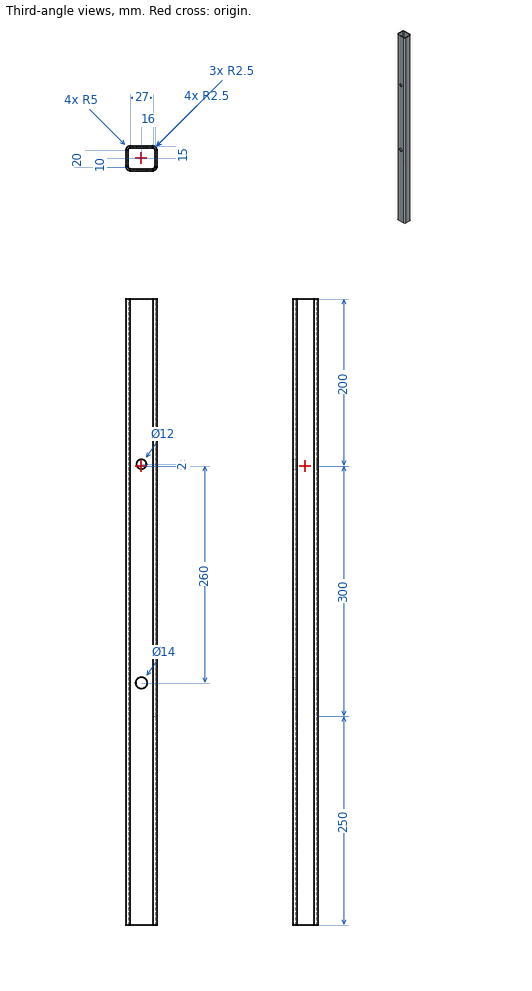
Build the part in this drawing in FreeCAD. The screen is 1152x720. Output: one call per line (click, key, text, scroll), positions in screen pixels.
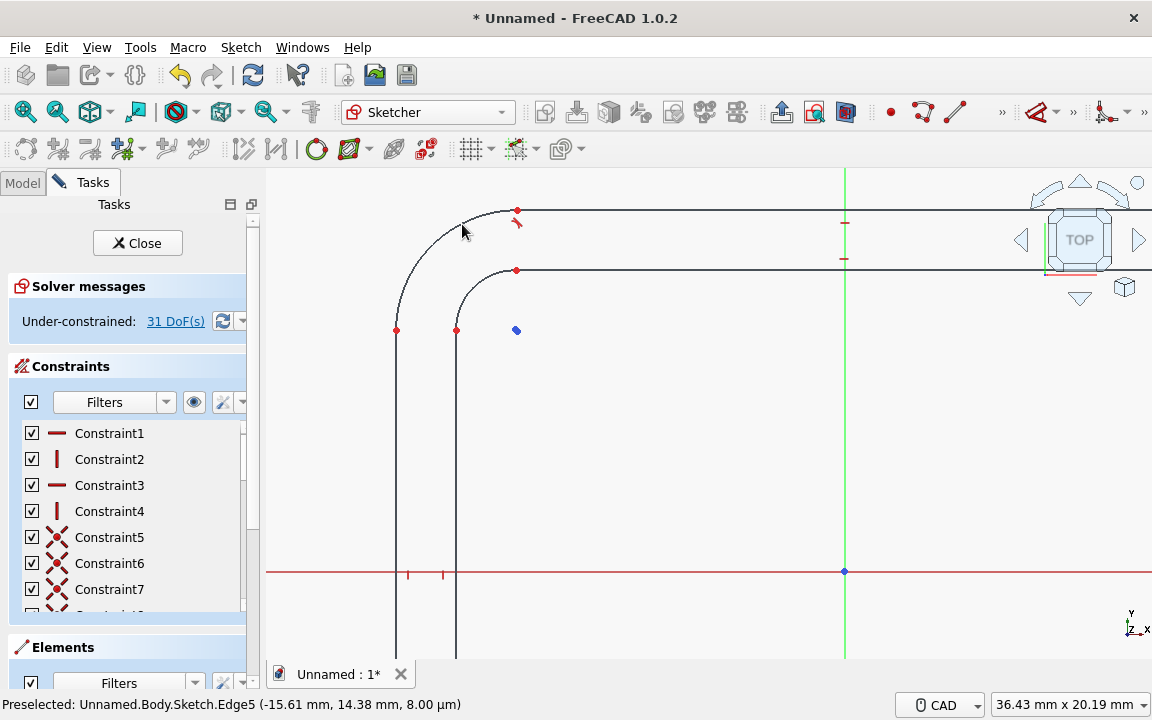
click(976, 210)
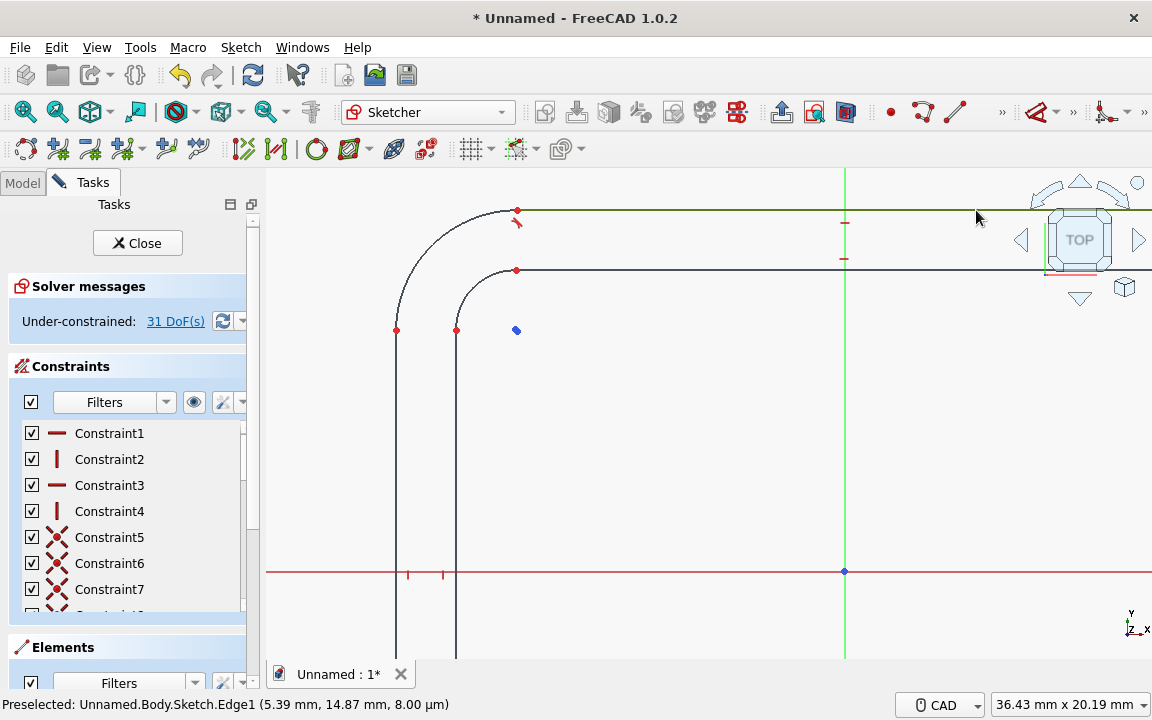
scroll(474, 284, down, 4)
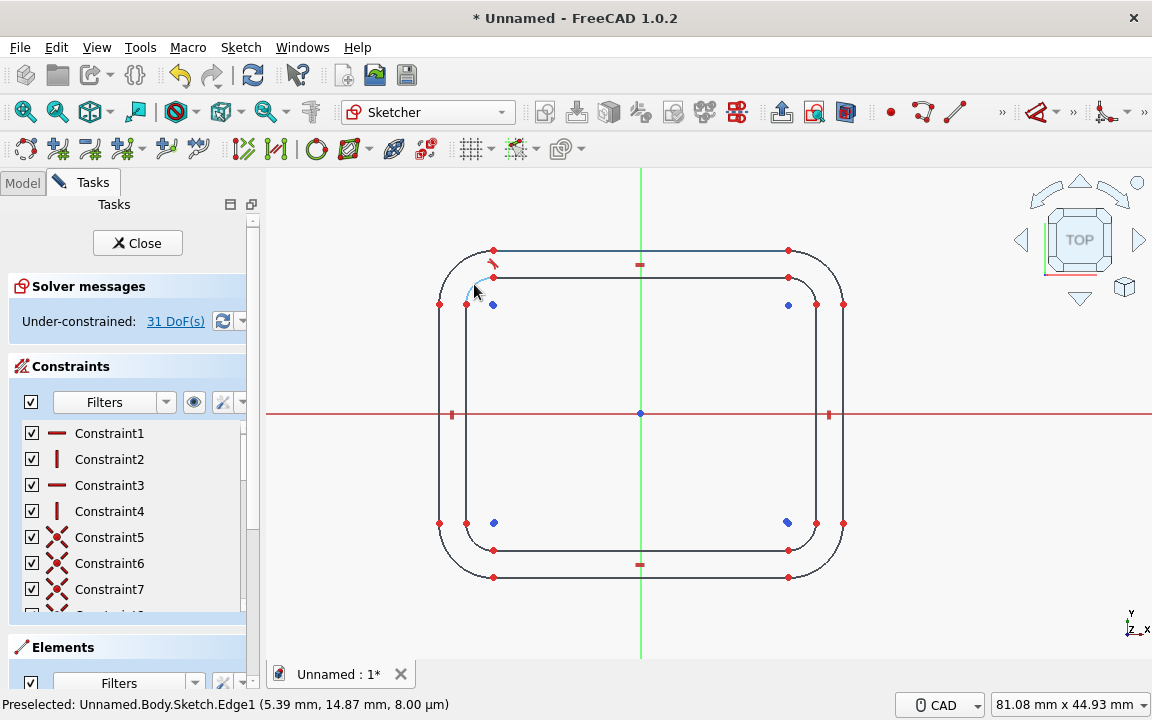
click(837, 280)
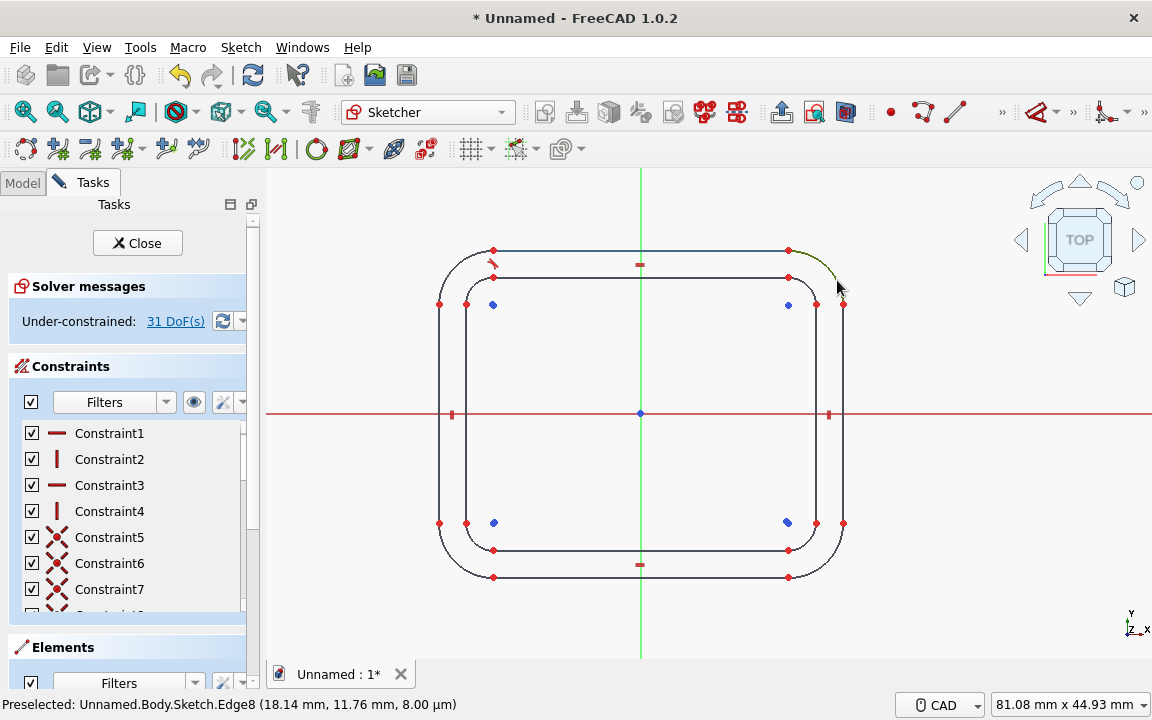
key(t)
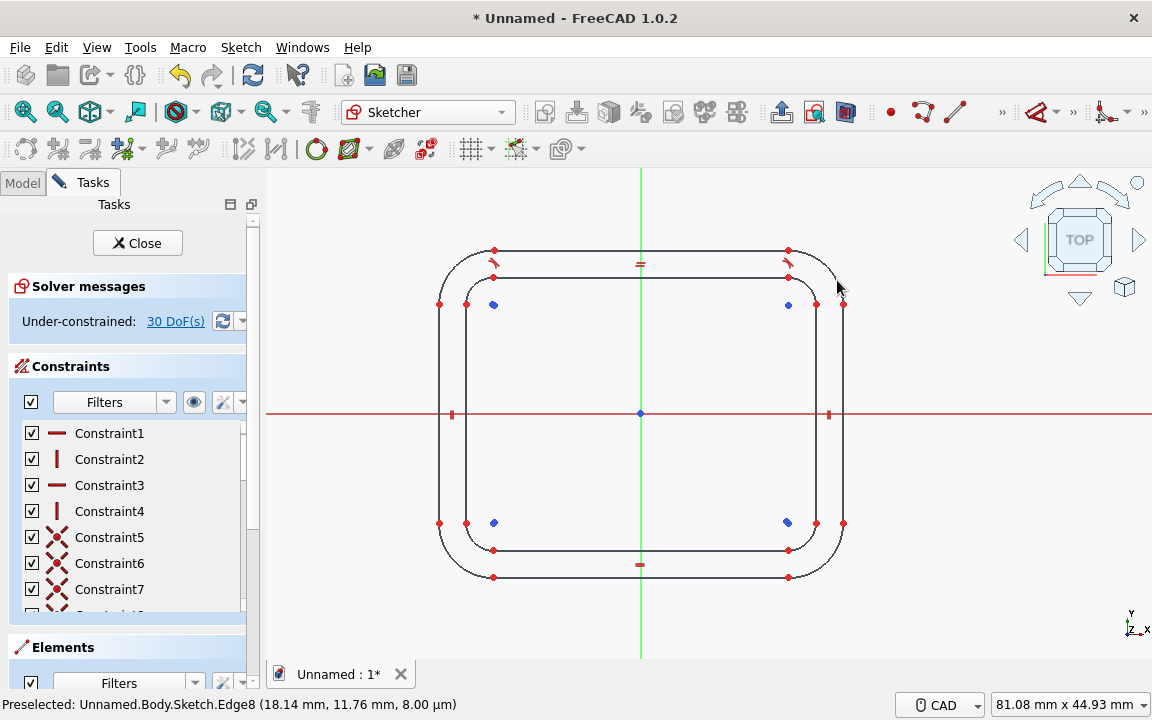
click(439, 371)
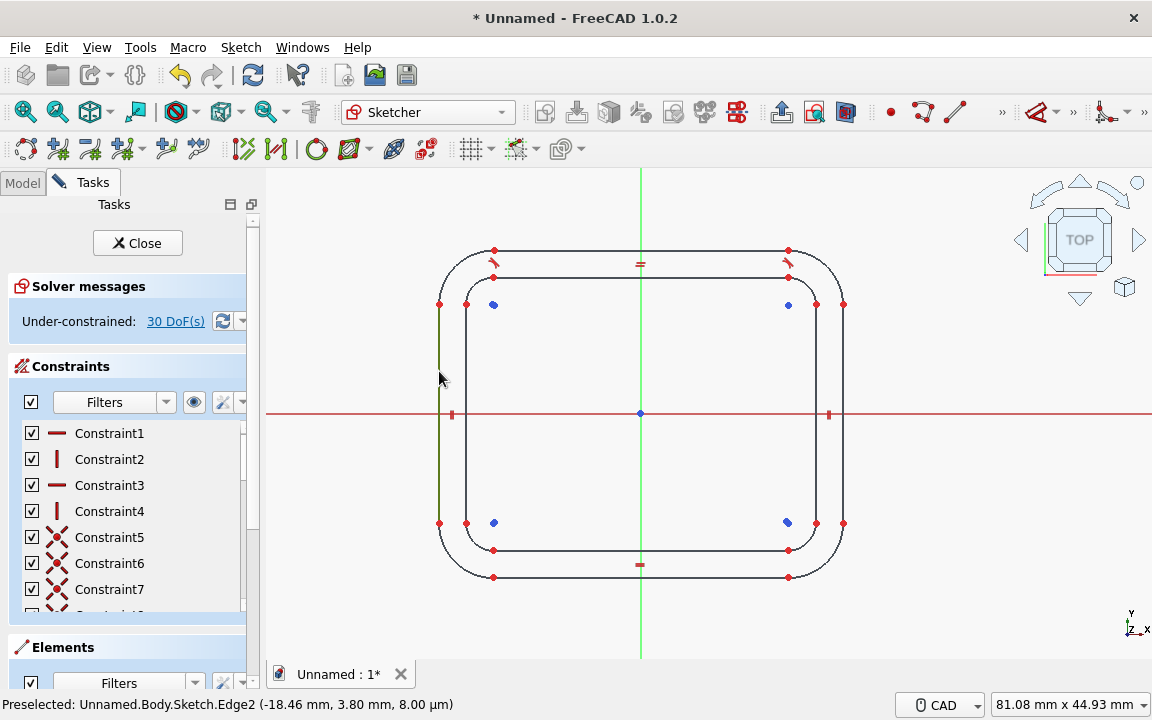
click(469, 257)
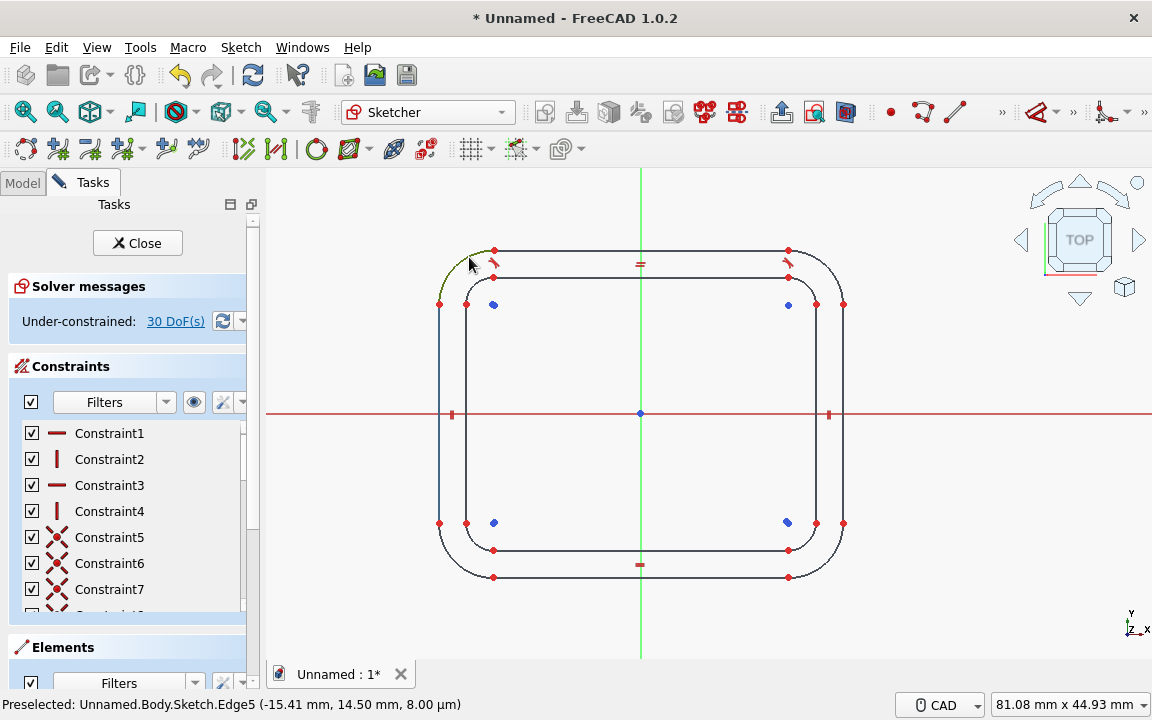
key(t)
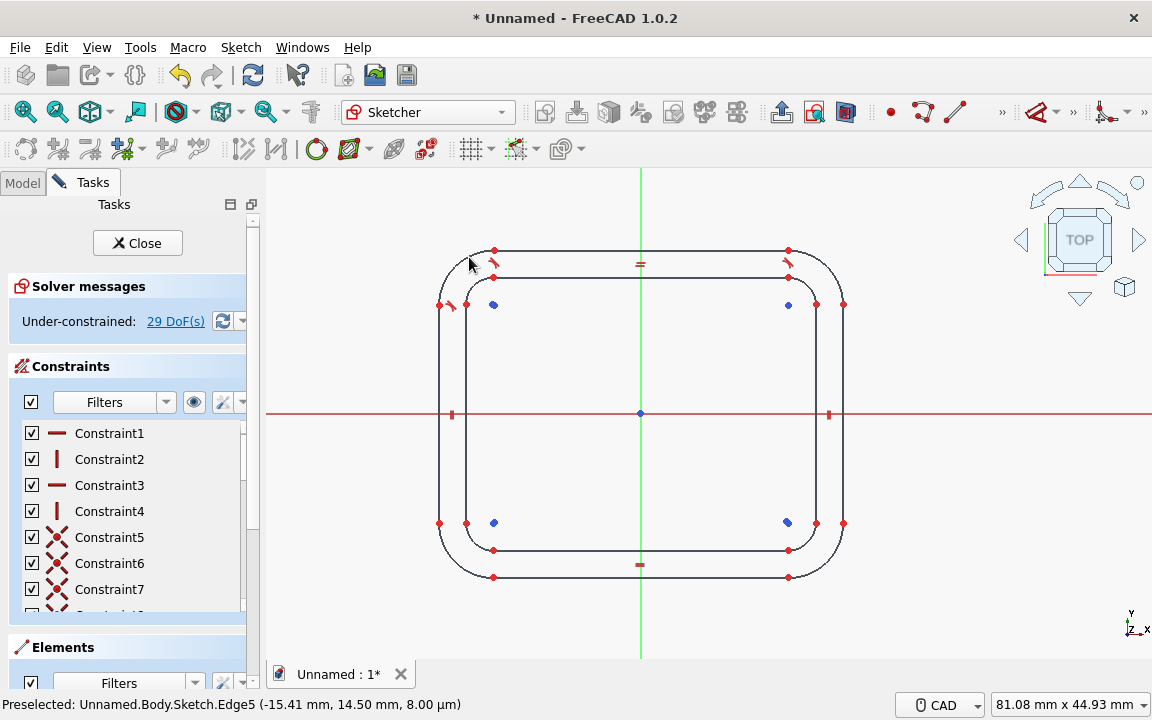
click(439, 371)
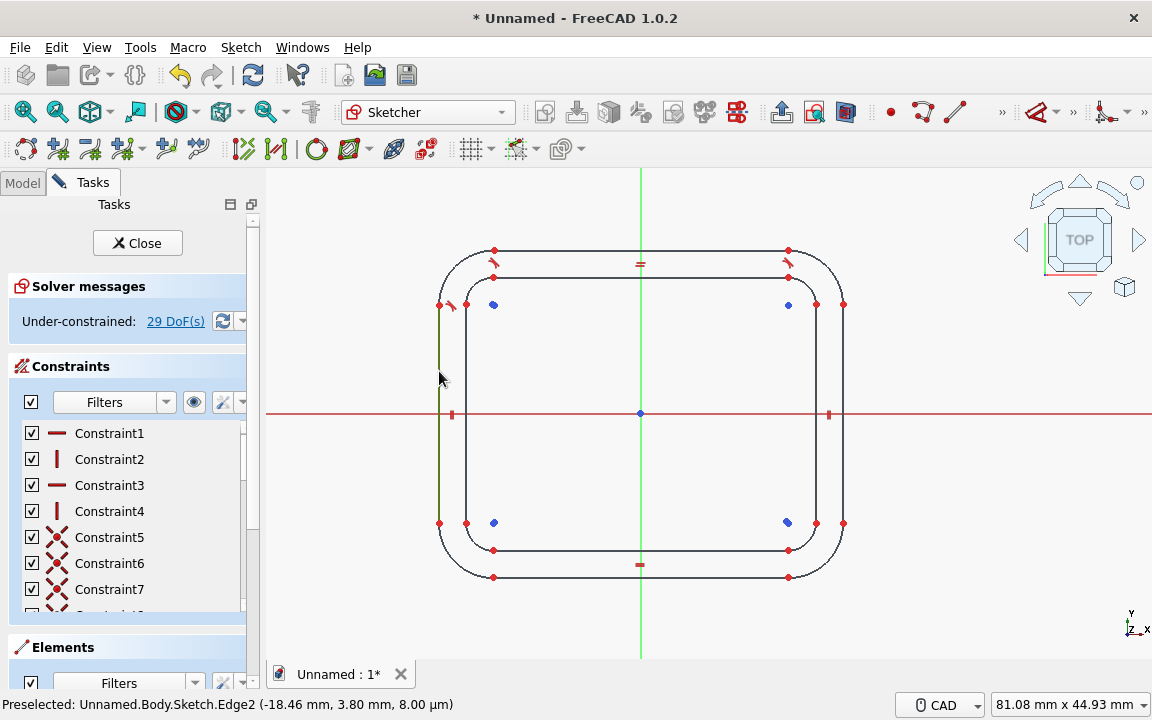
click(445, 548)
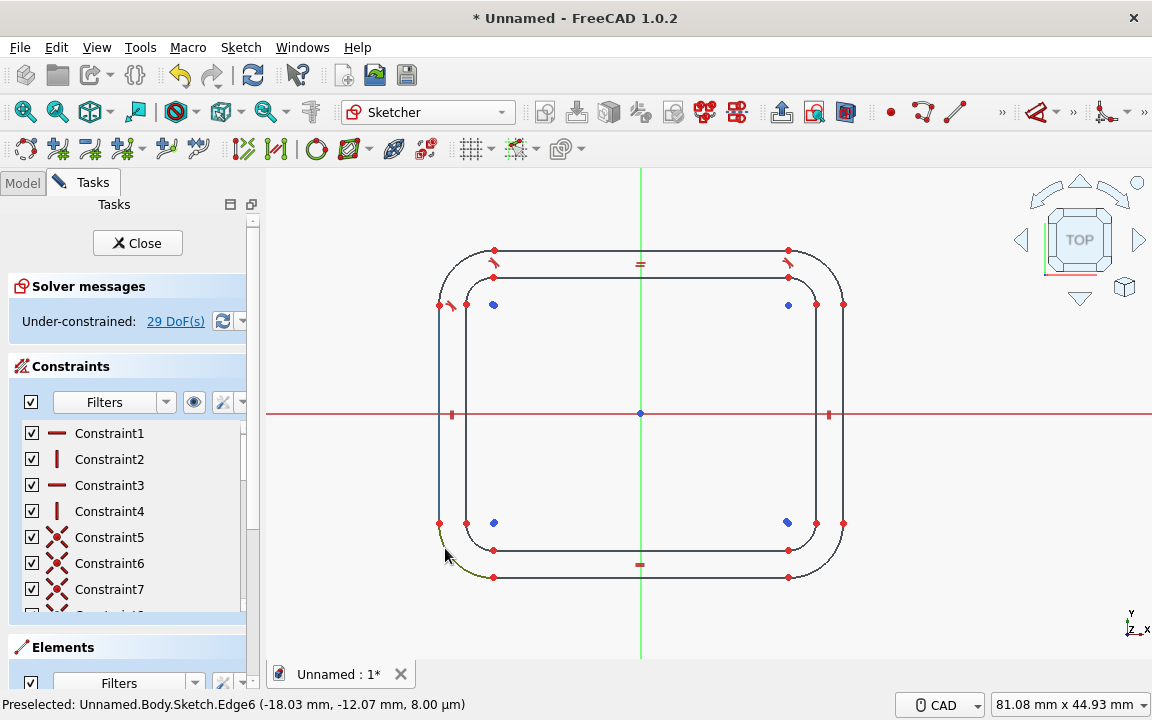
key(t)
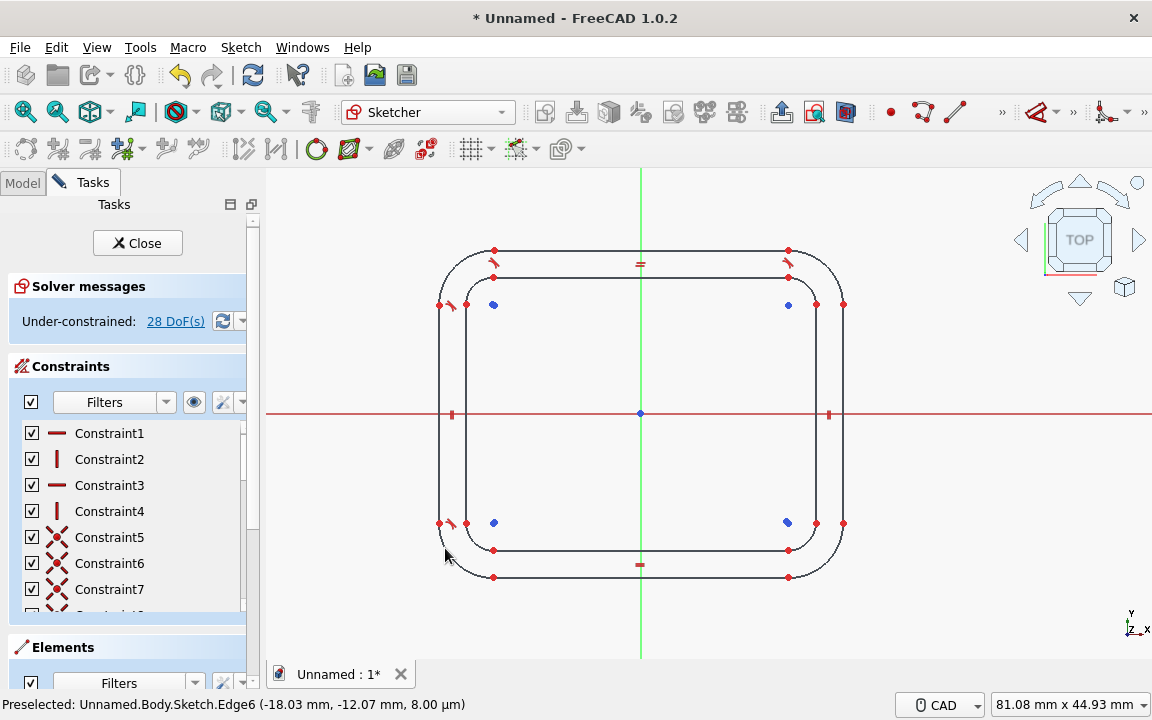
click(582, 578)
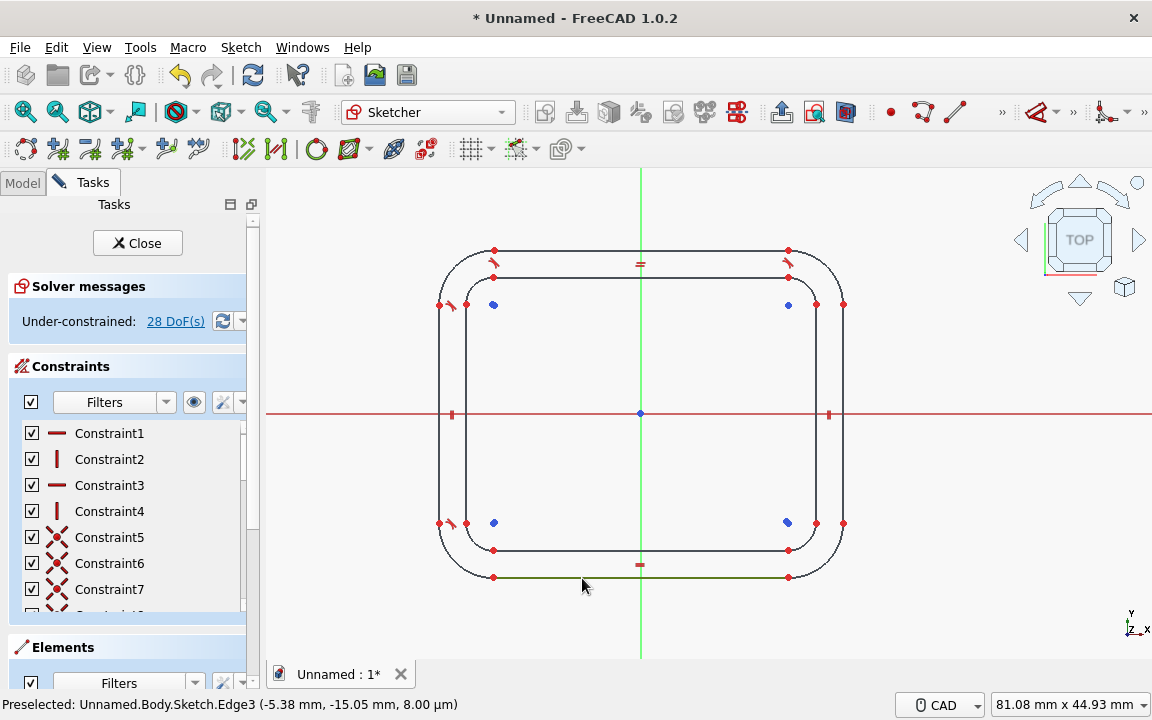
click(445, 548)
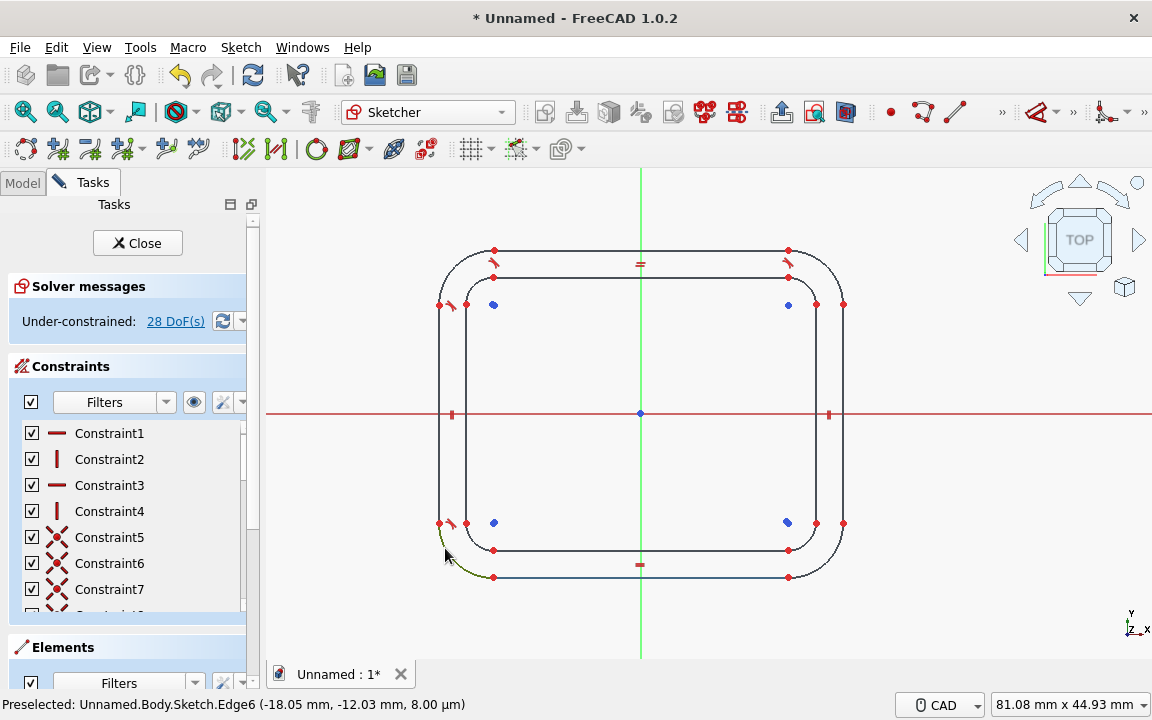
key(t)